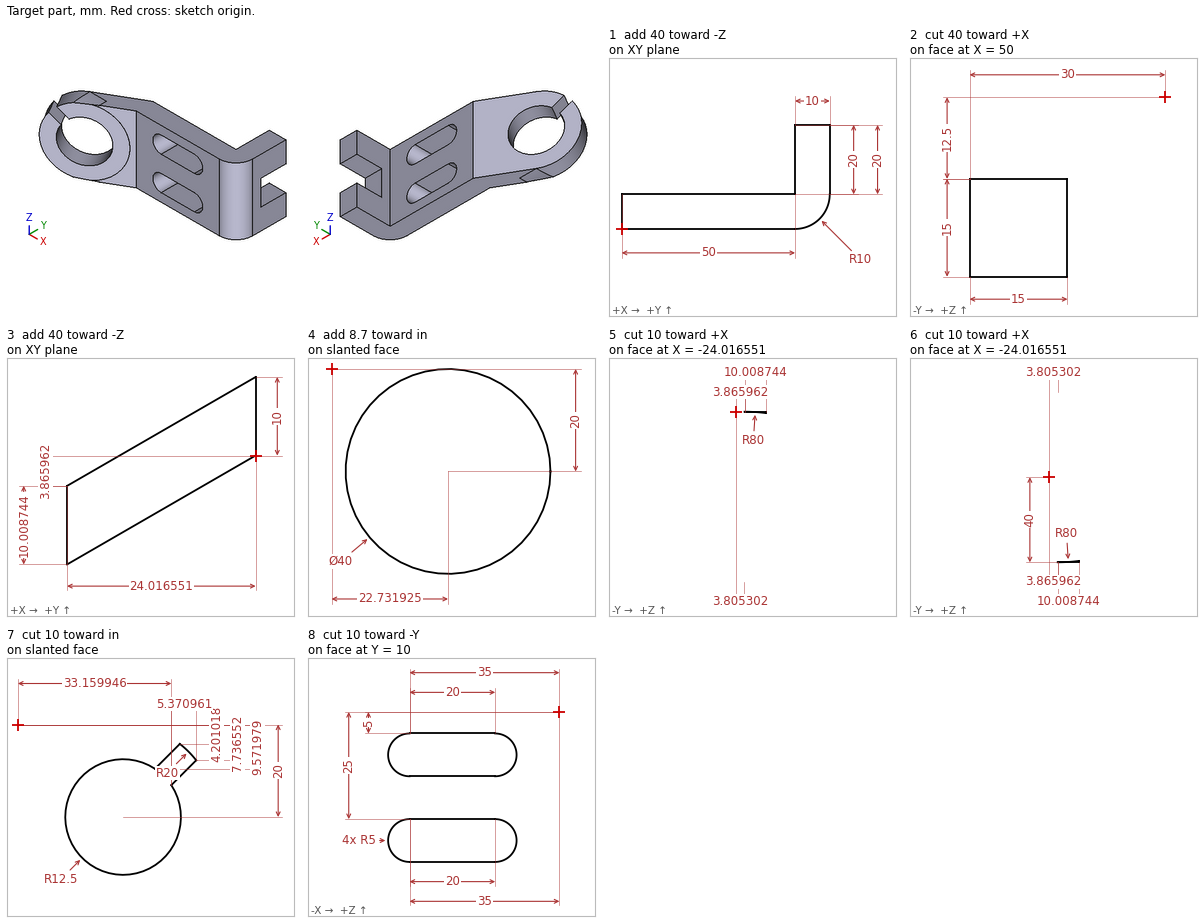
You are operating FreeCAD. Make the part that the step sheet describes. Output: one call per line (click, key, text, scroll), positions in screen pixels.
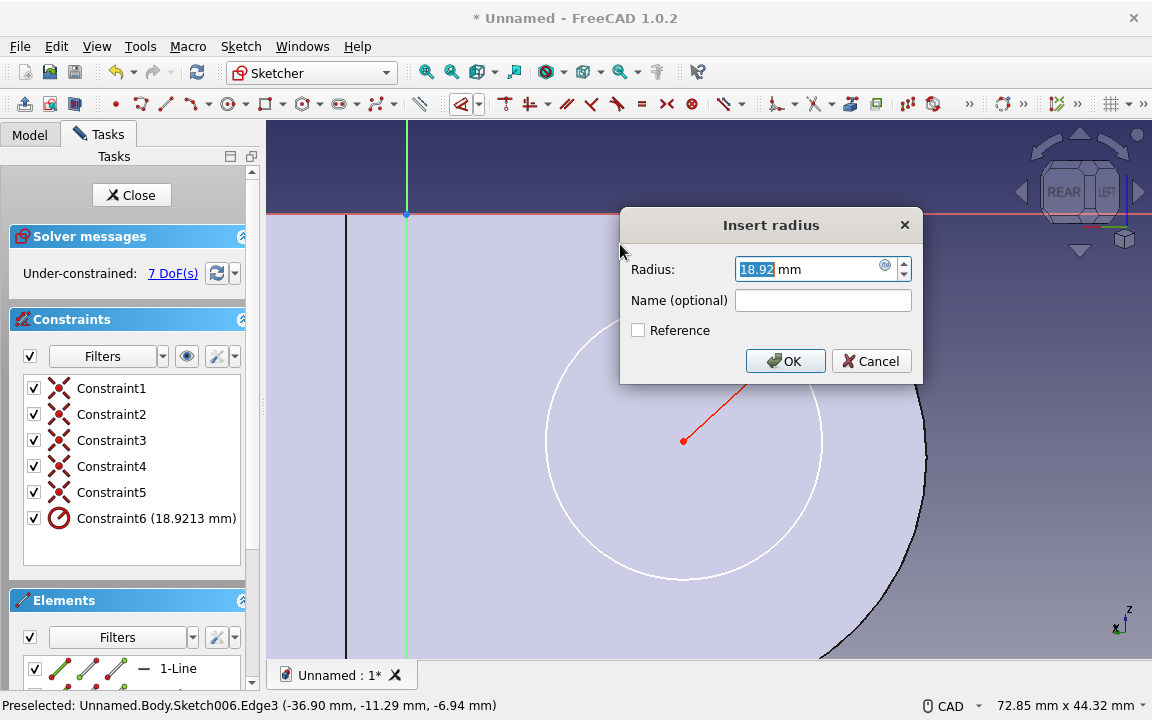
text(20)
key(Return)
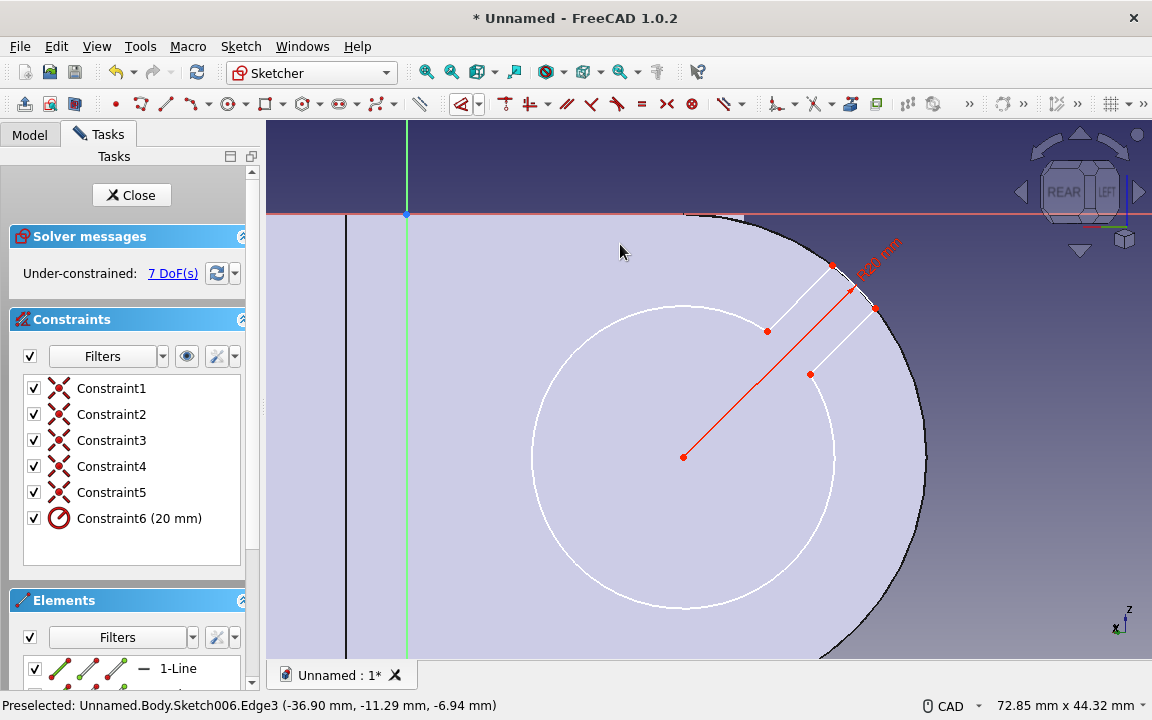
click(544, 399)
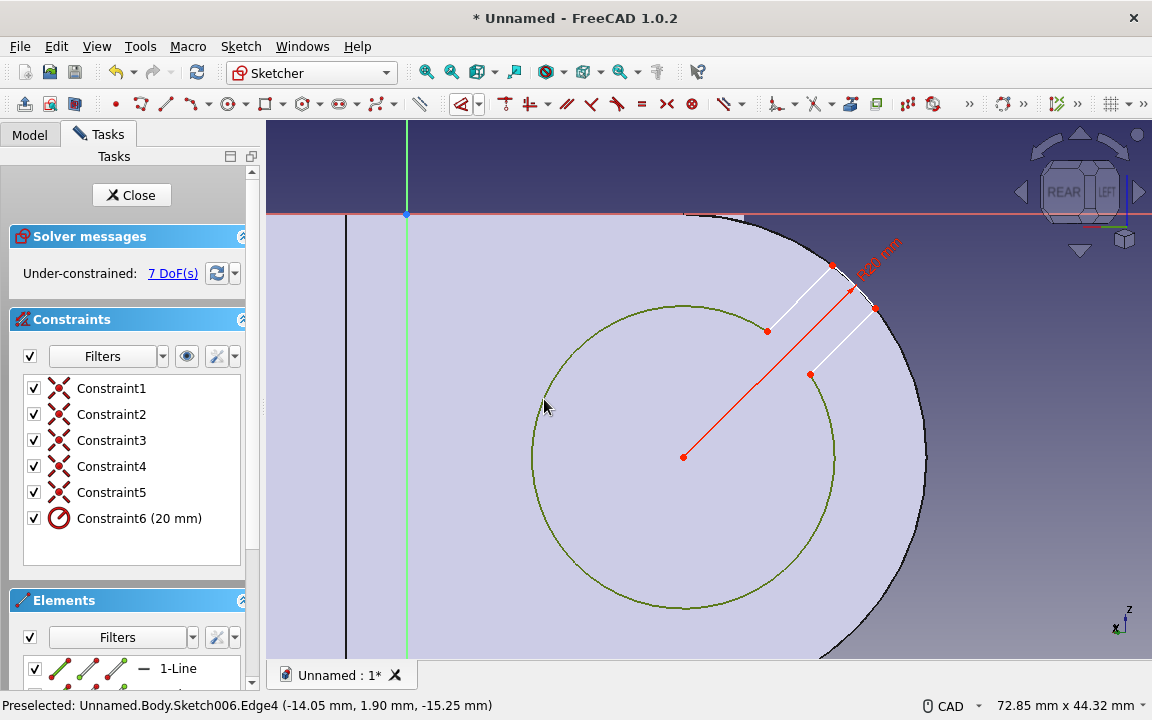
key(k)
key(r)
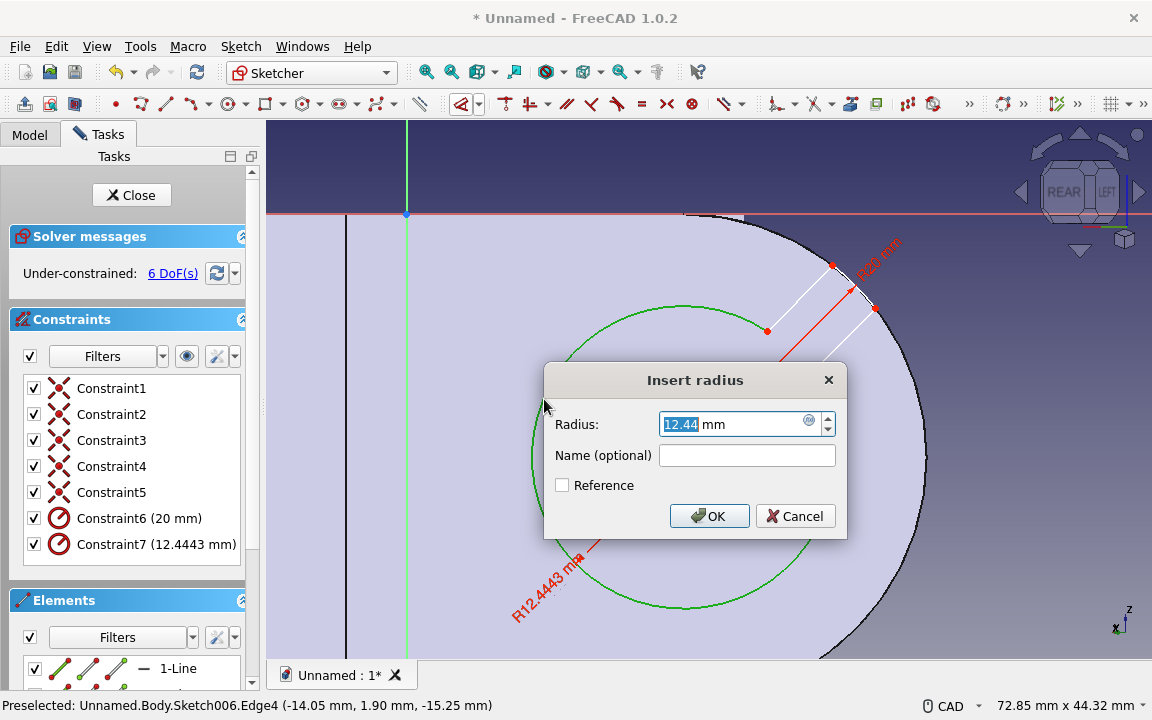
text(12.5)
key(Return)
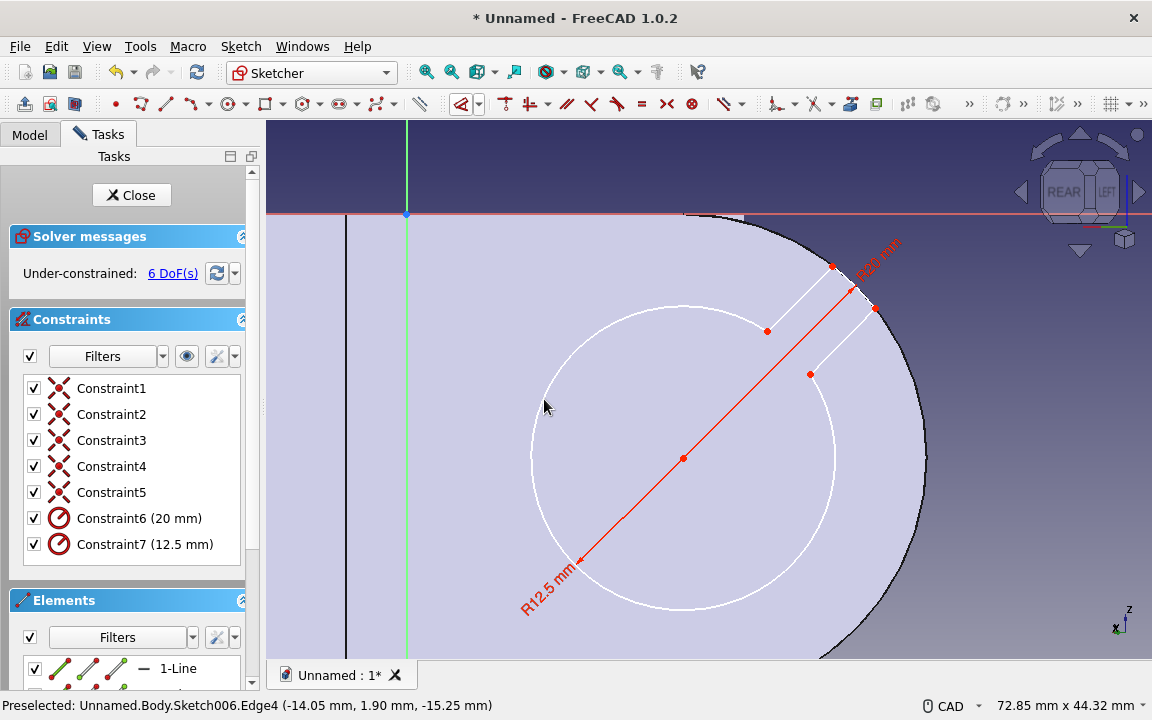
click(683, 458)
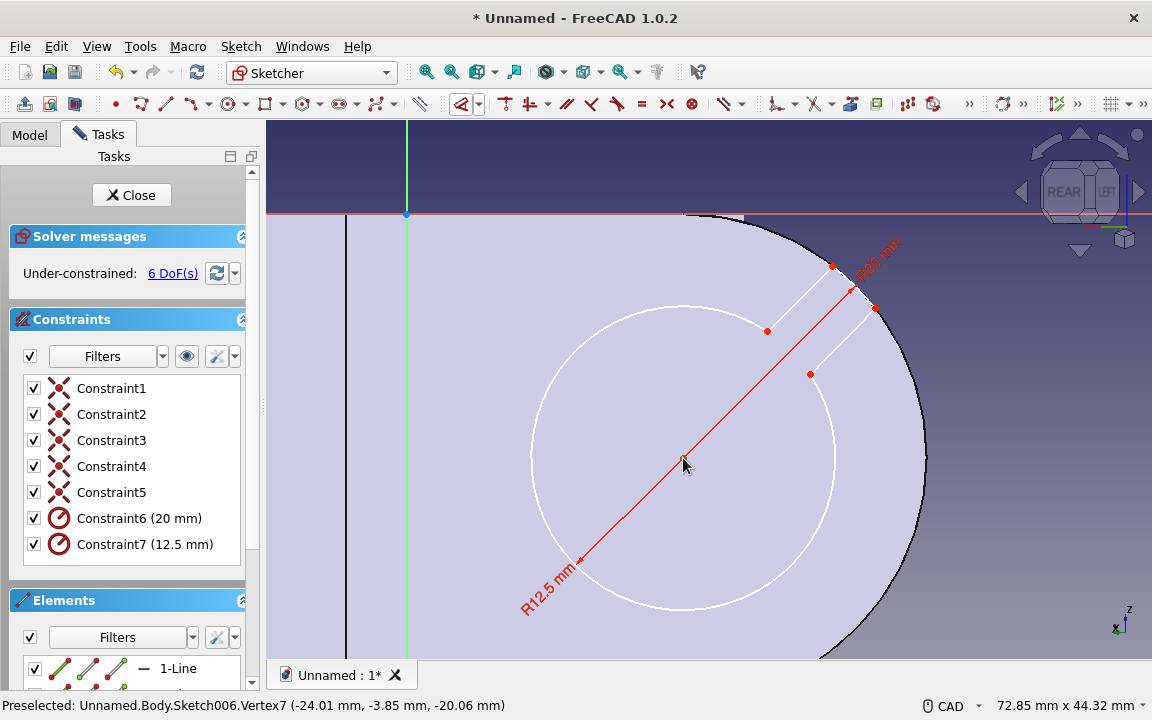
click(478, 104)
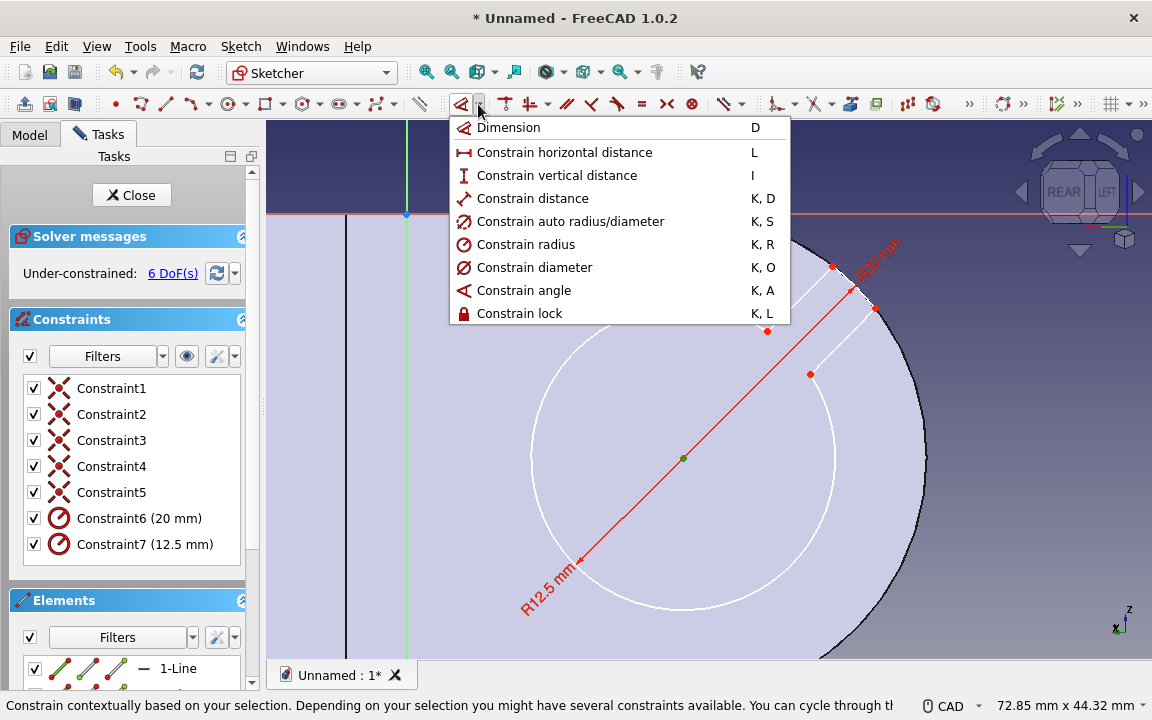
click(620, 176)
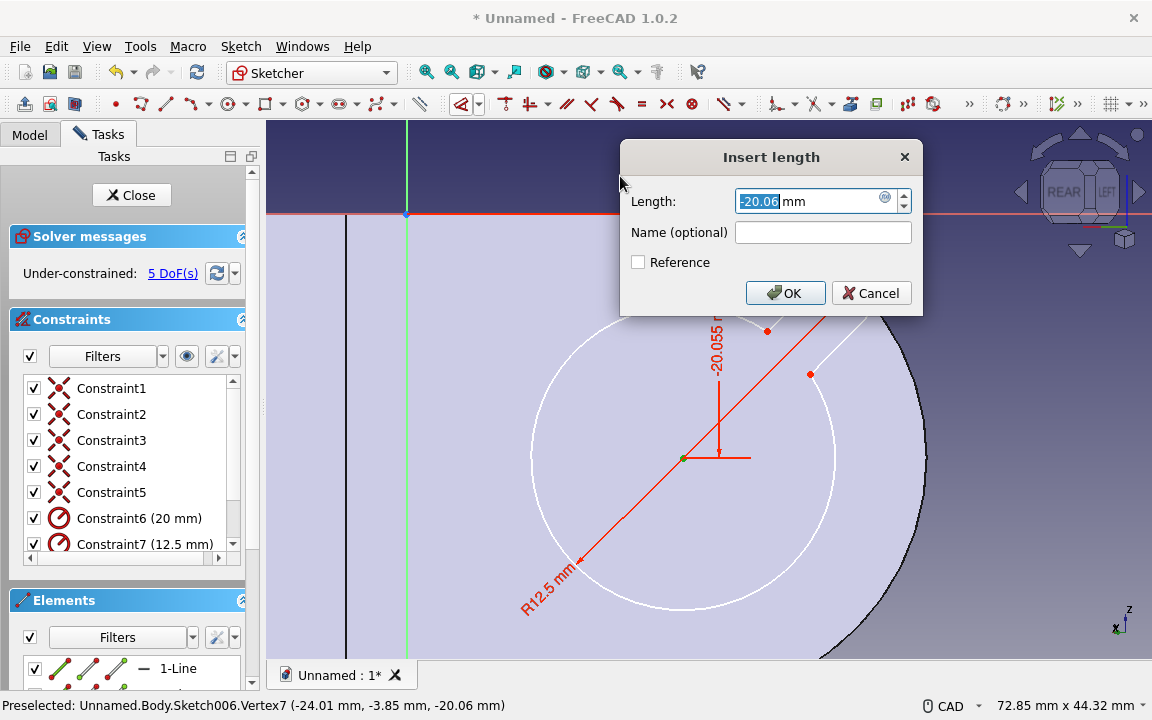
text(-20)
key(Return)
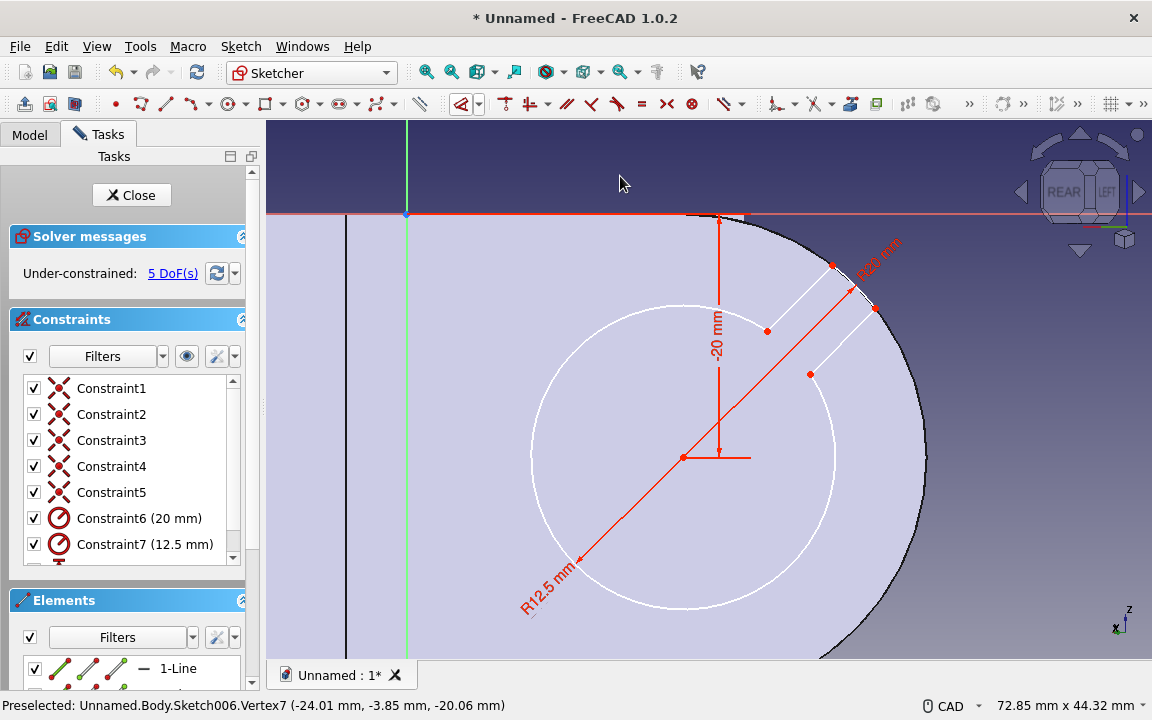
click(876, 309)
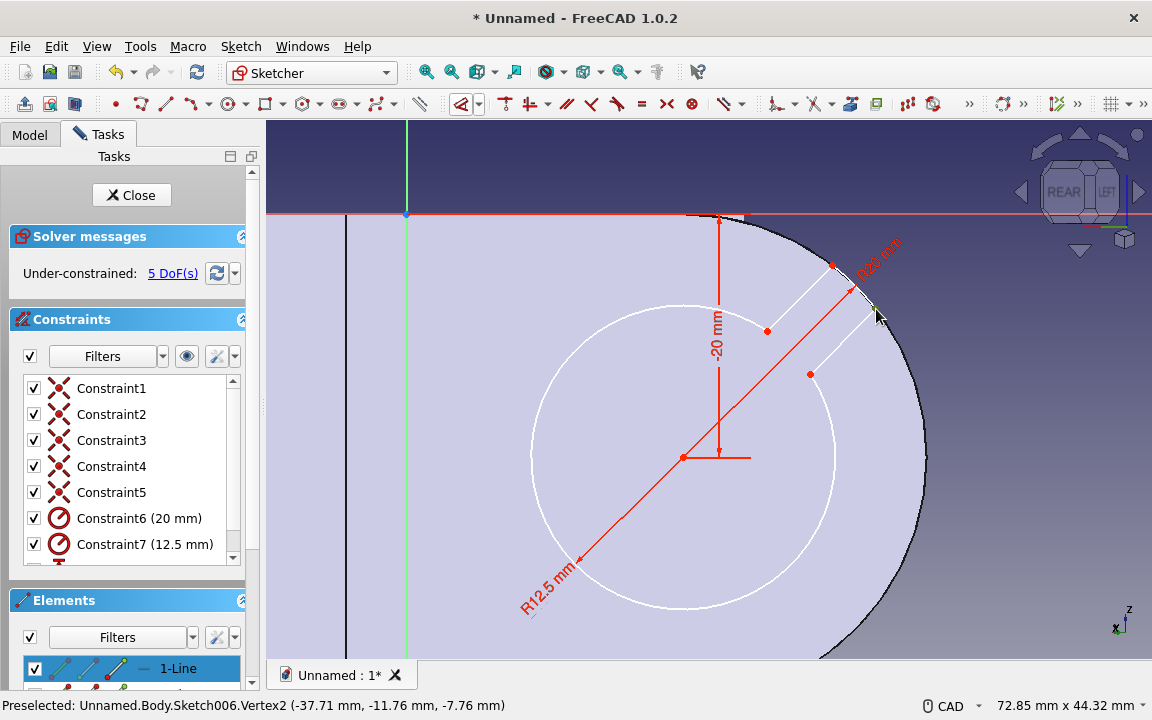
key(i)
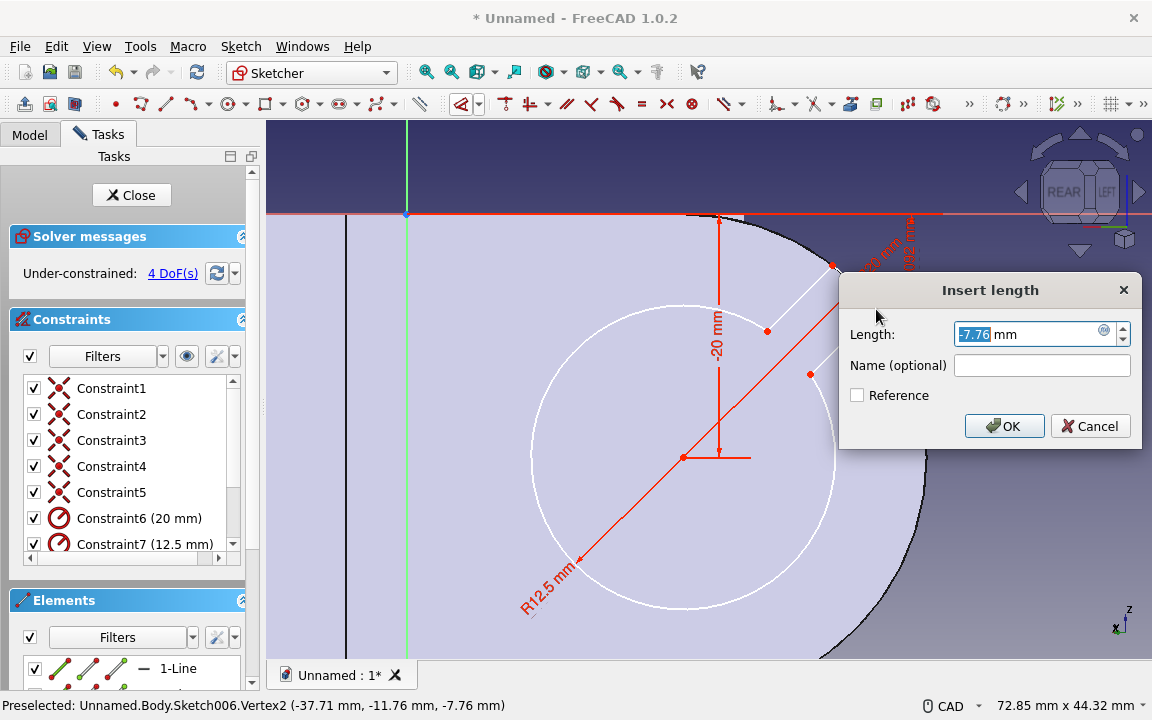
text(-7.736552)
key(Return)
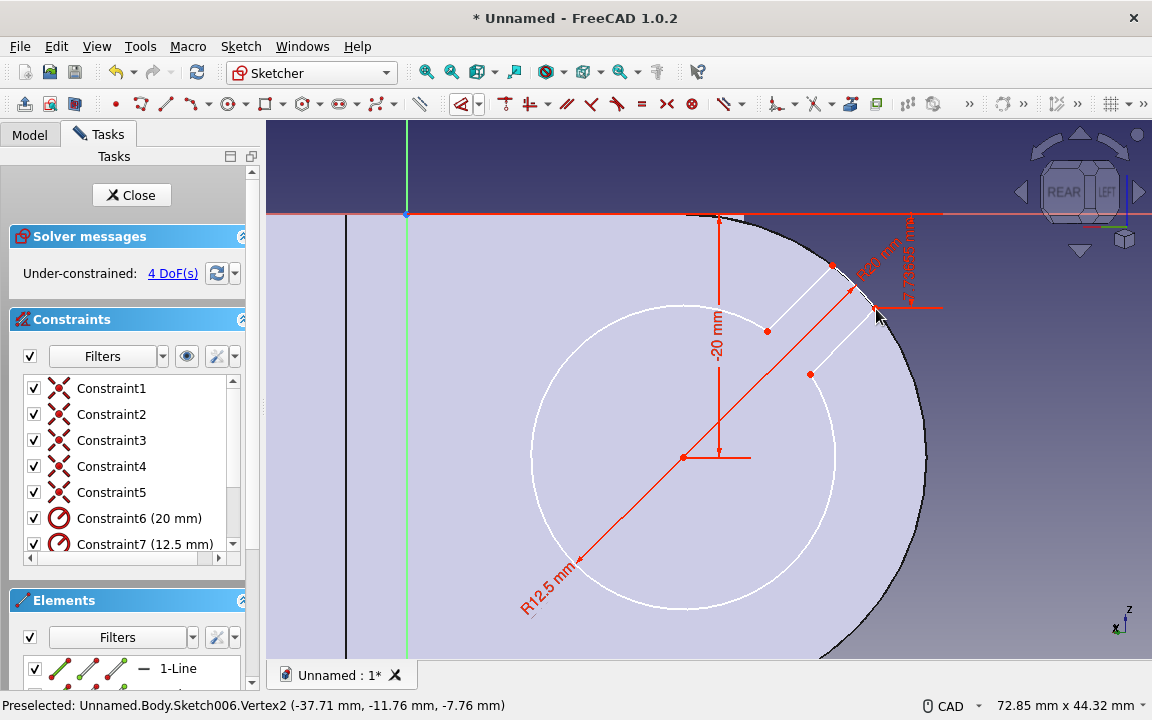
click(833, 266)